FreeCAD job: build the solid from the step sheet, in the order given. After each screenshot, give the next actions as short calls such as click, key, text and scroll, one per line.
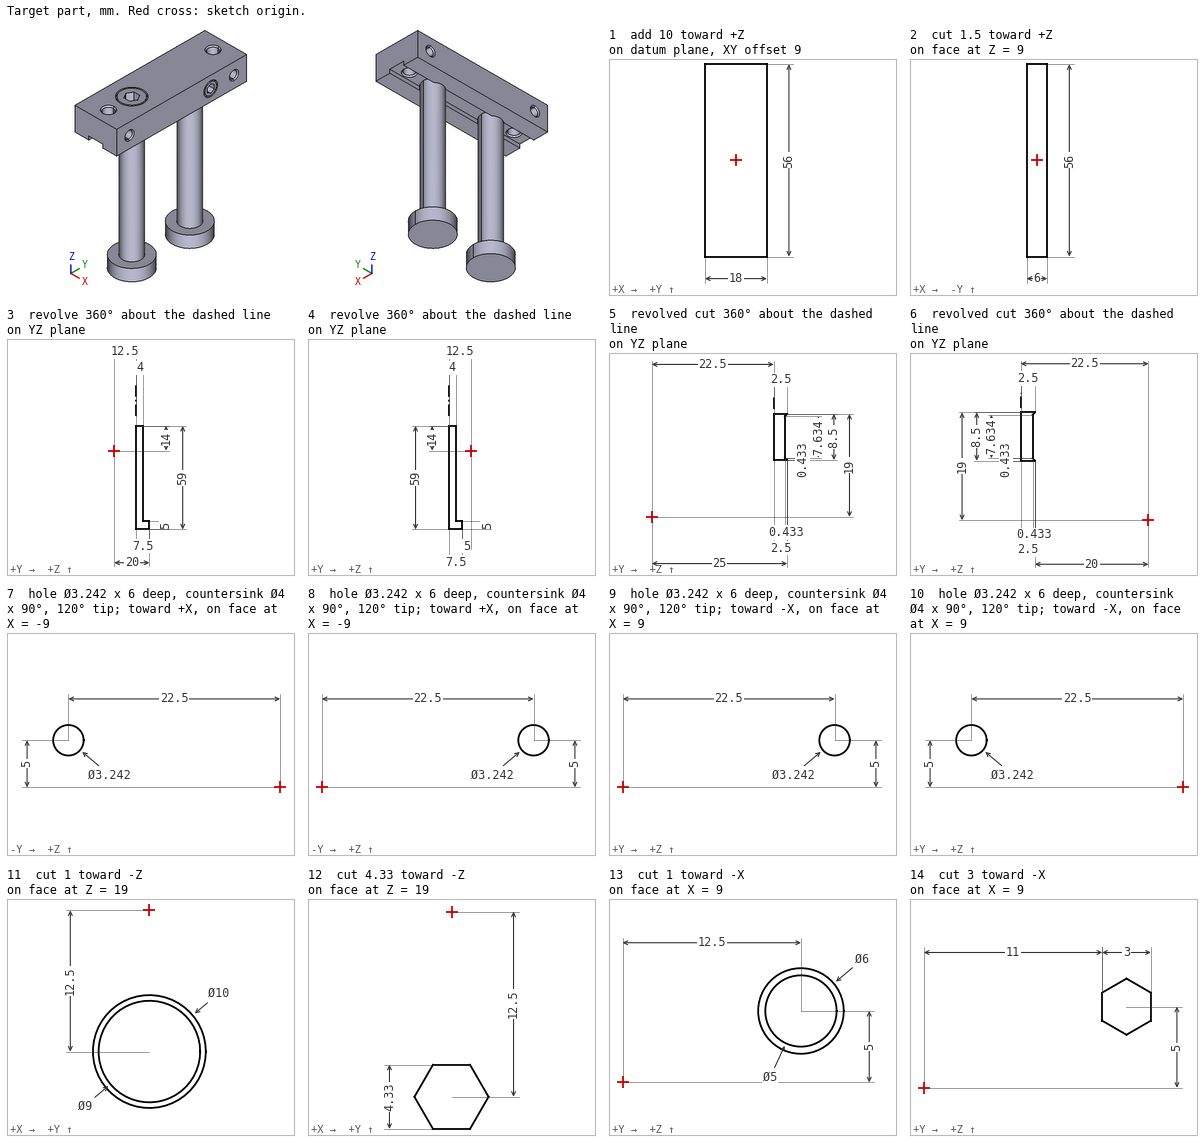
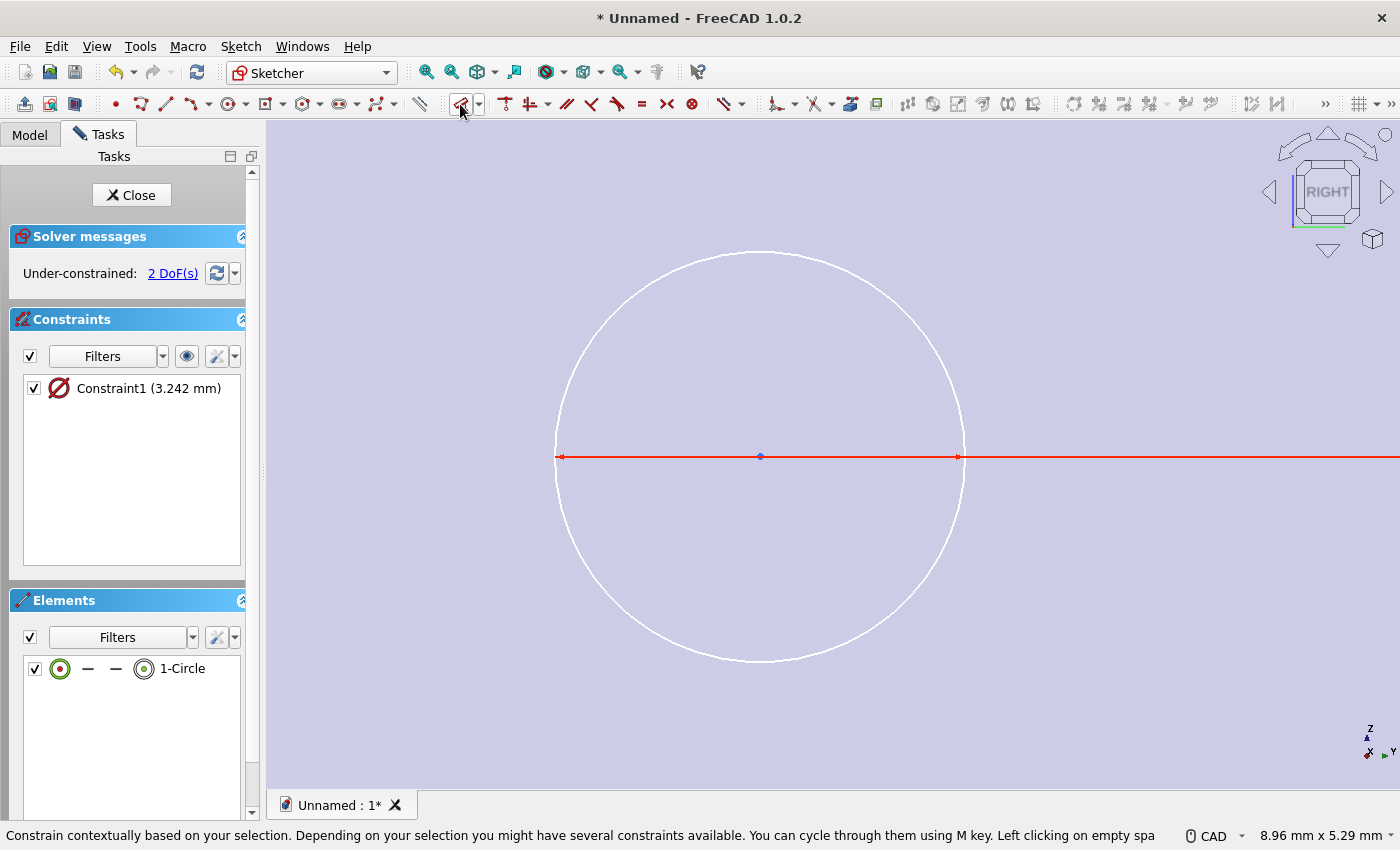
click(760, 457)
click(726, 609)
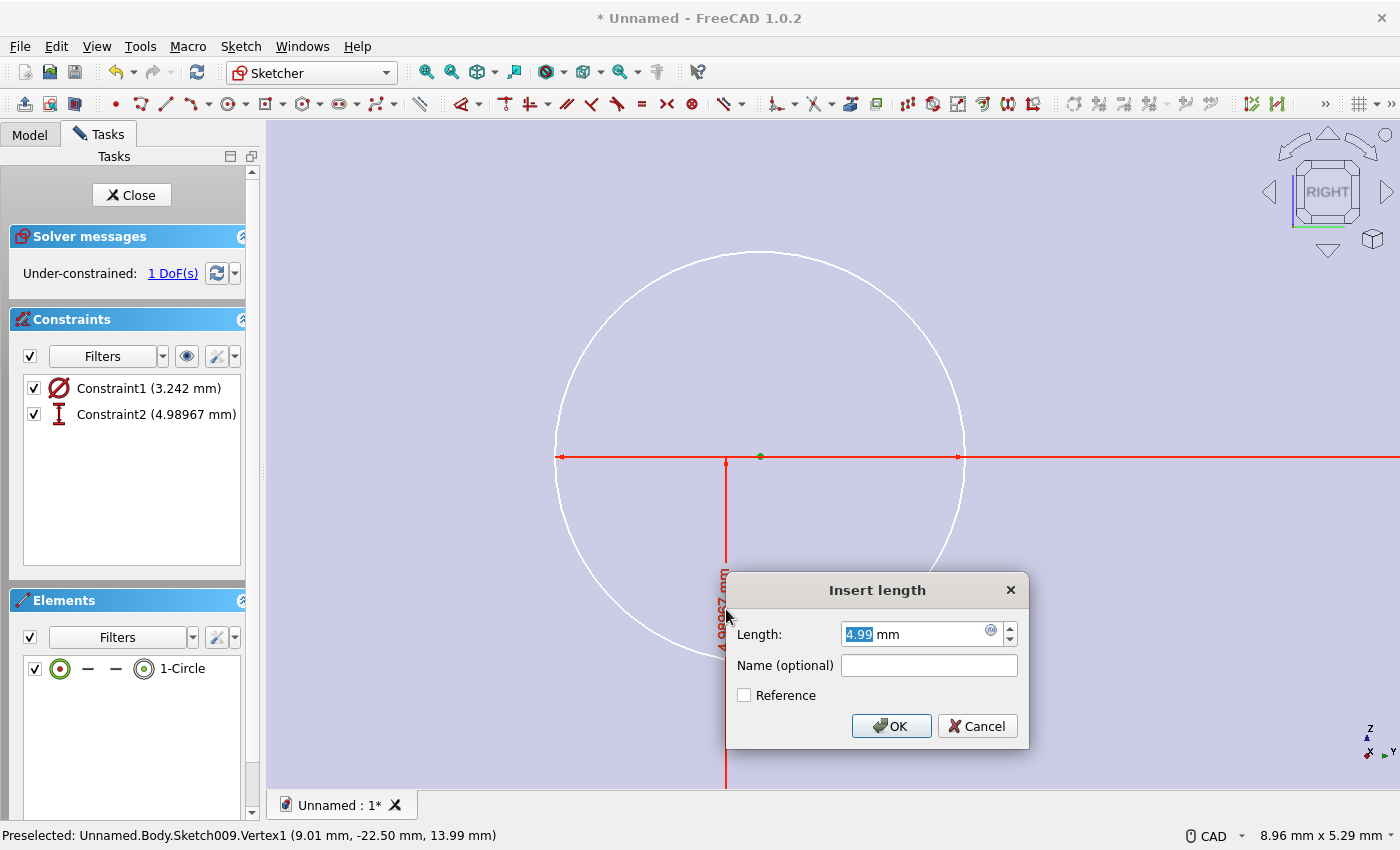
text(5)
key(Return)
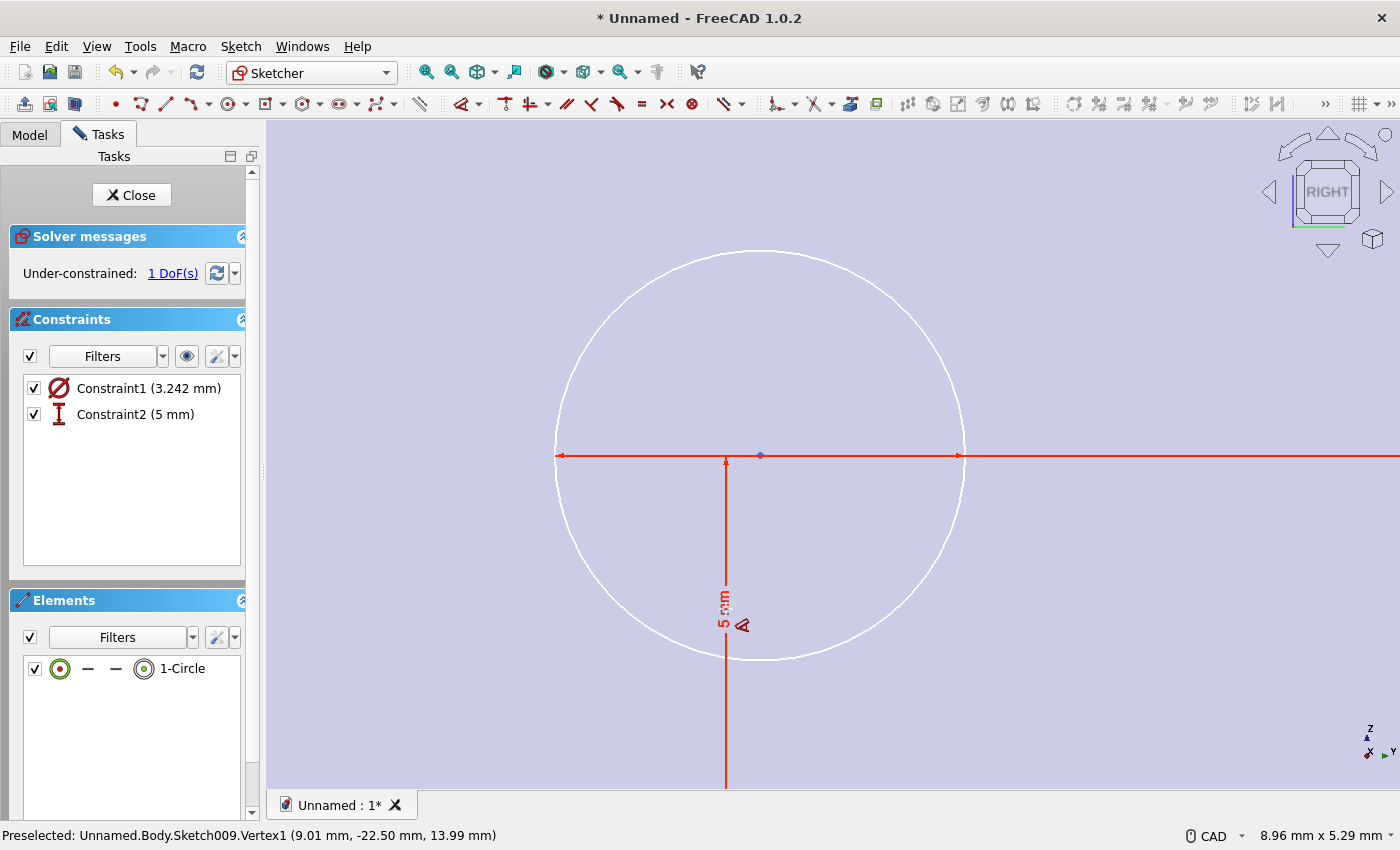
click(760, 456)
click(998, 422)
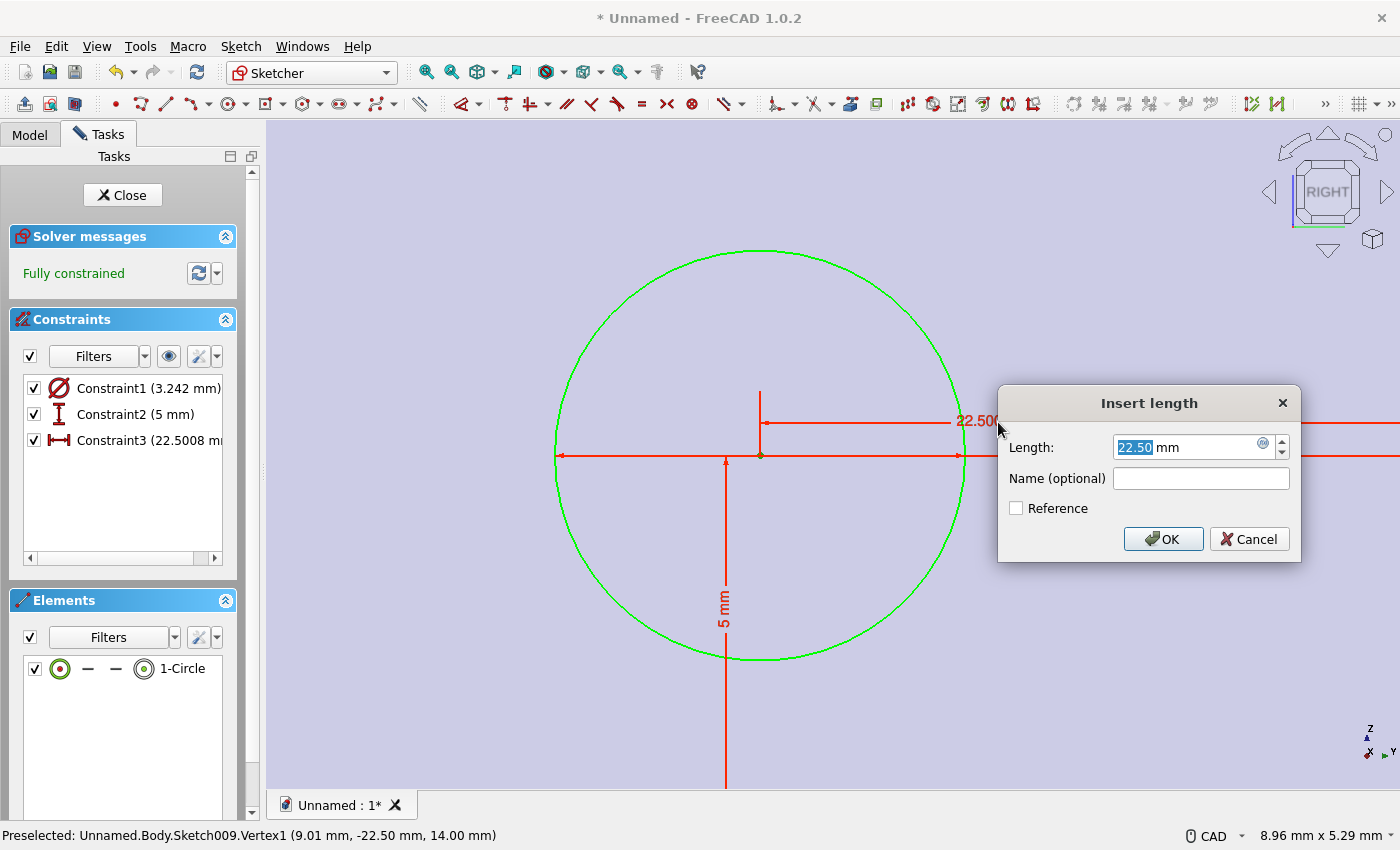
text(22.5)
key(Return)
key(Escape)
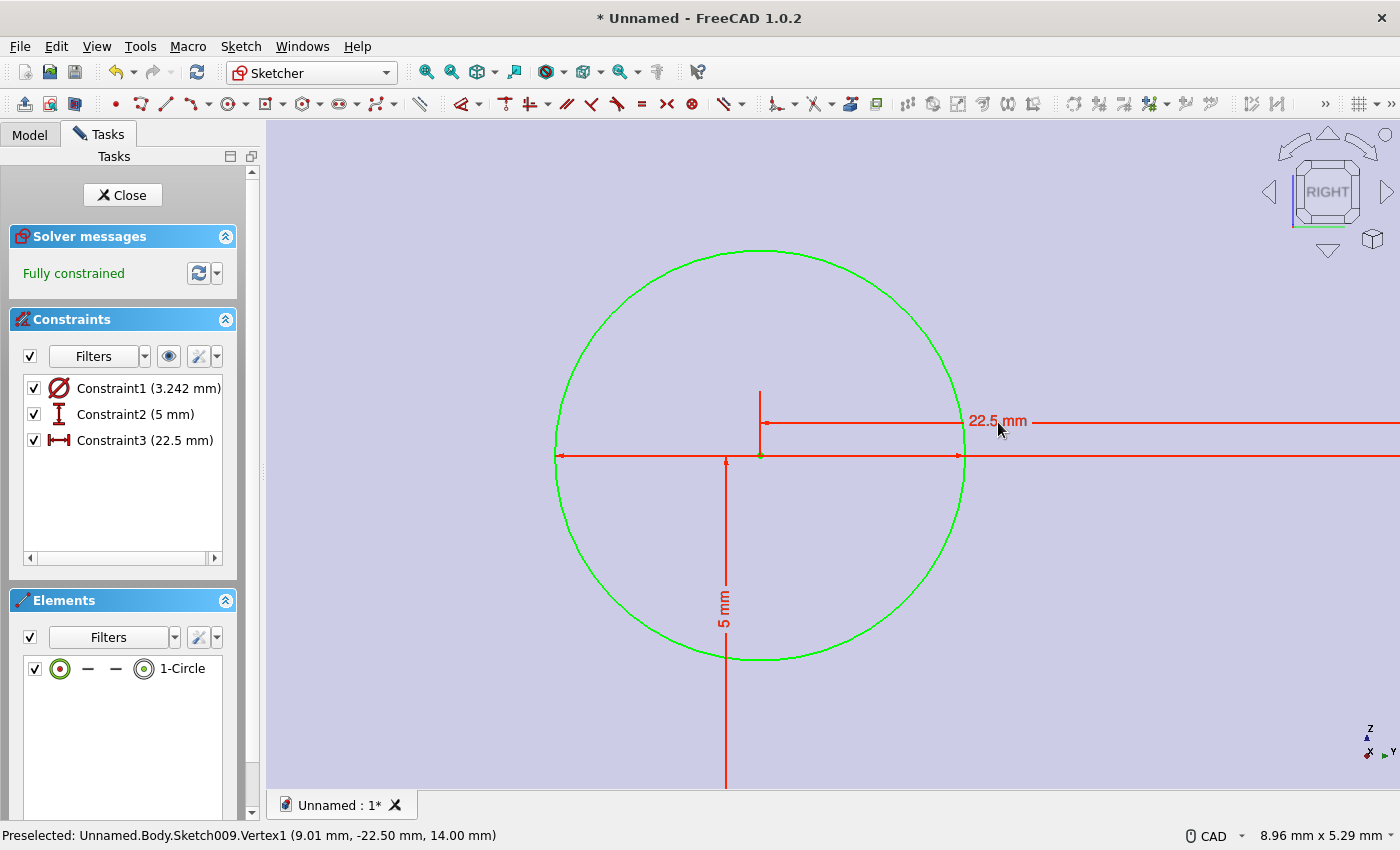
click(123, 195)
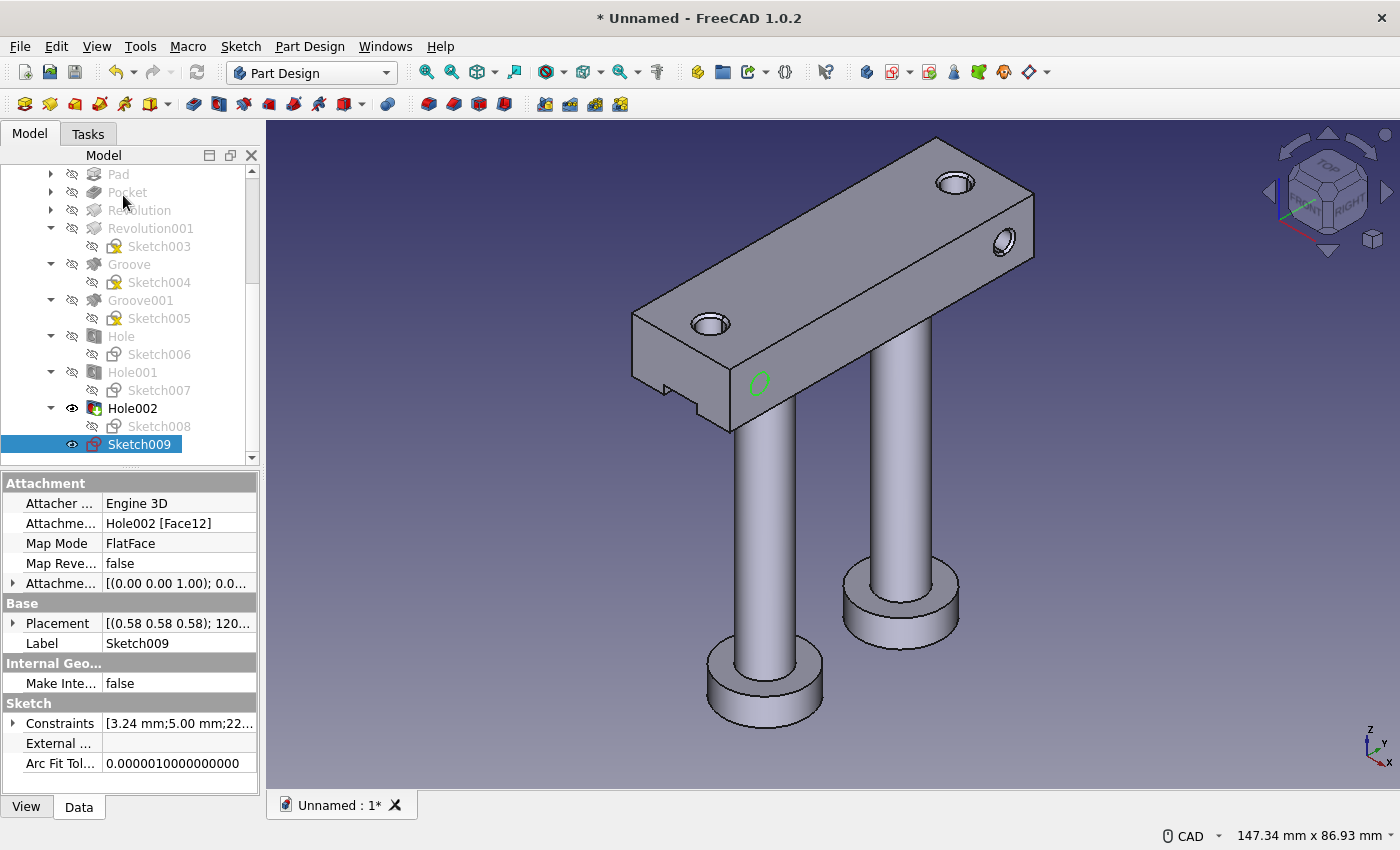
click(219, 104)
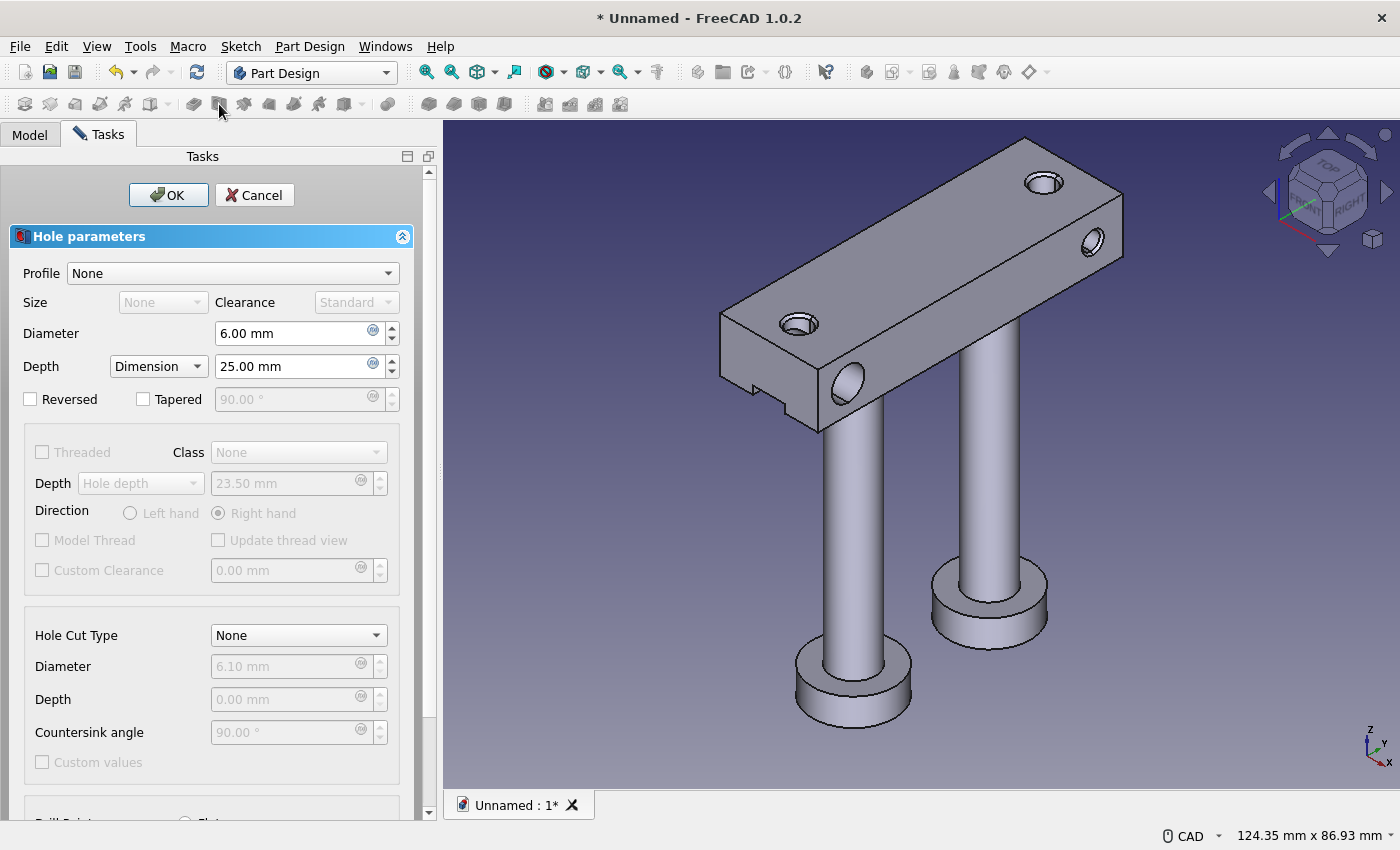
triple_click(300, 334)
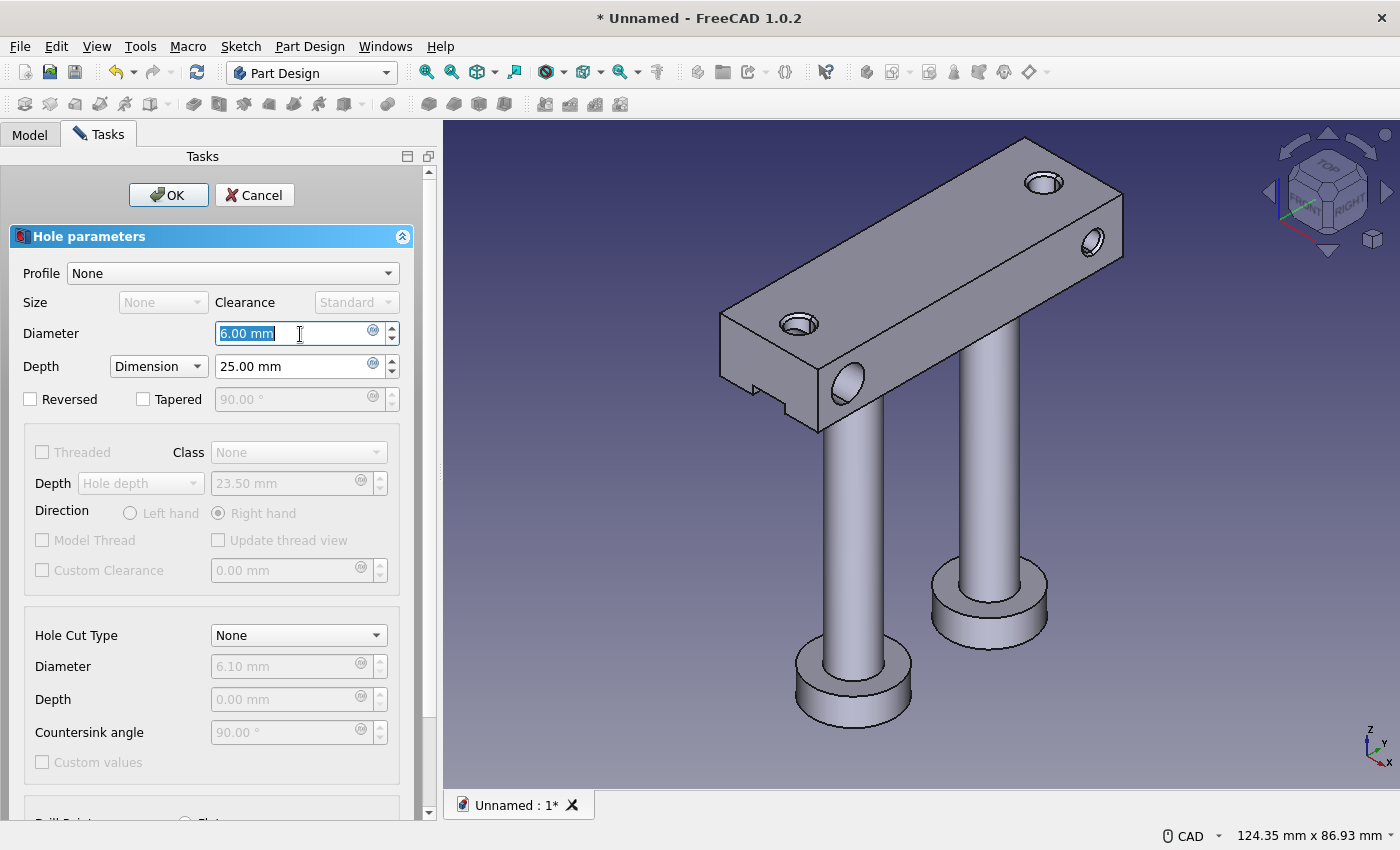
text(3.242)
key(Tab)